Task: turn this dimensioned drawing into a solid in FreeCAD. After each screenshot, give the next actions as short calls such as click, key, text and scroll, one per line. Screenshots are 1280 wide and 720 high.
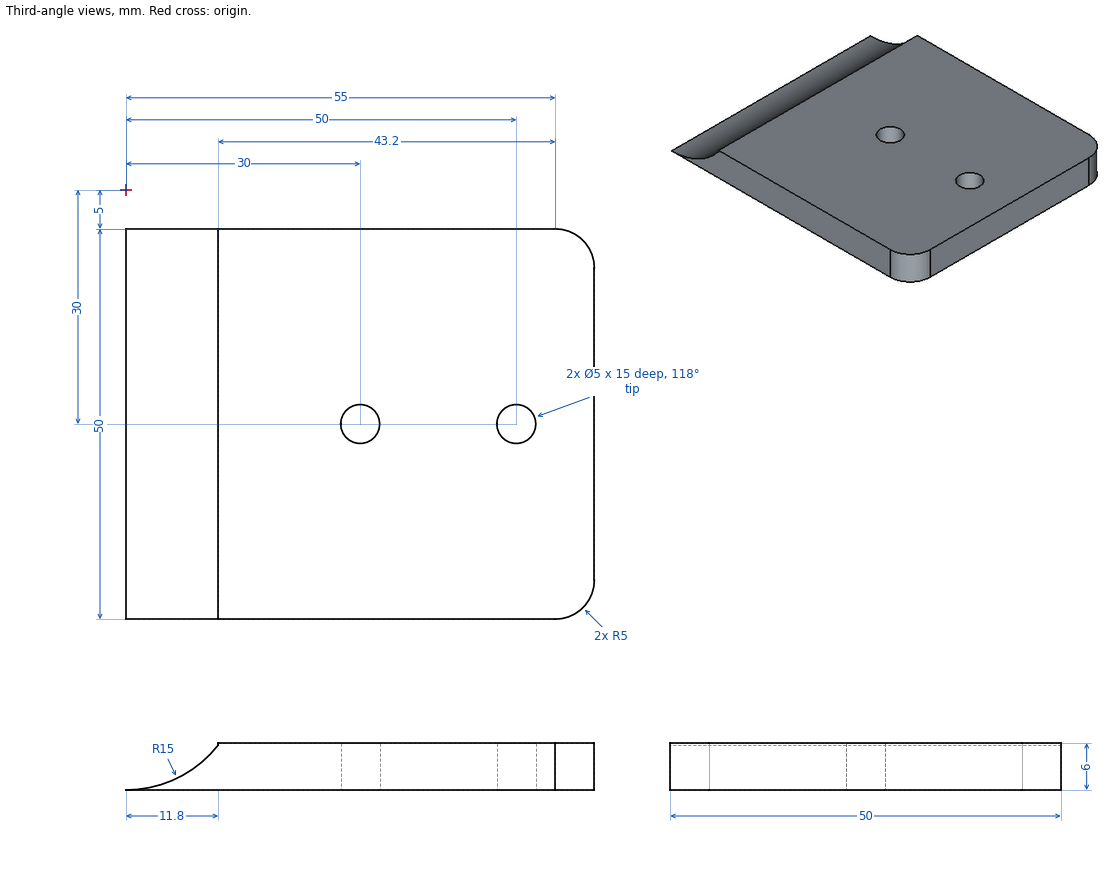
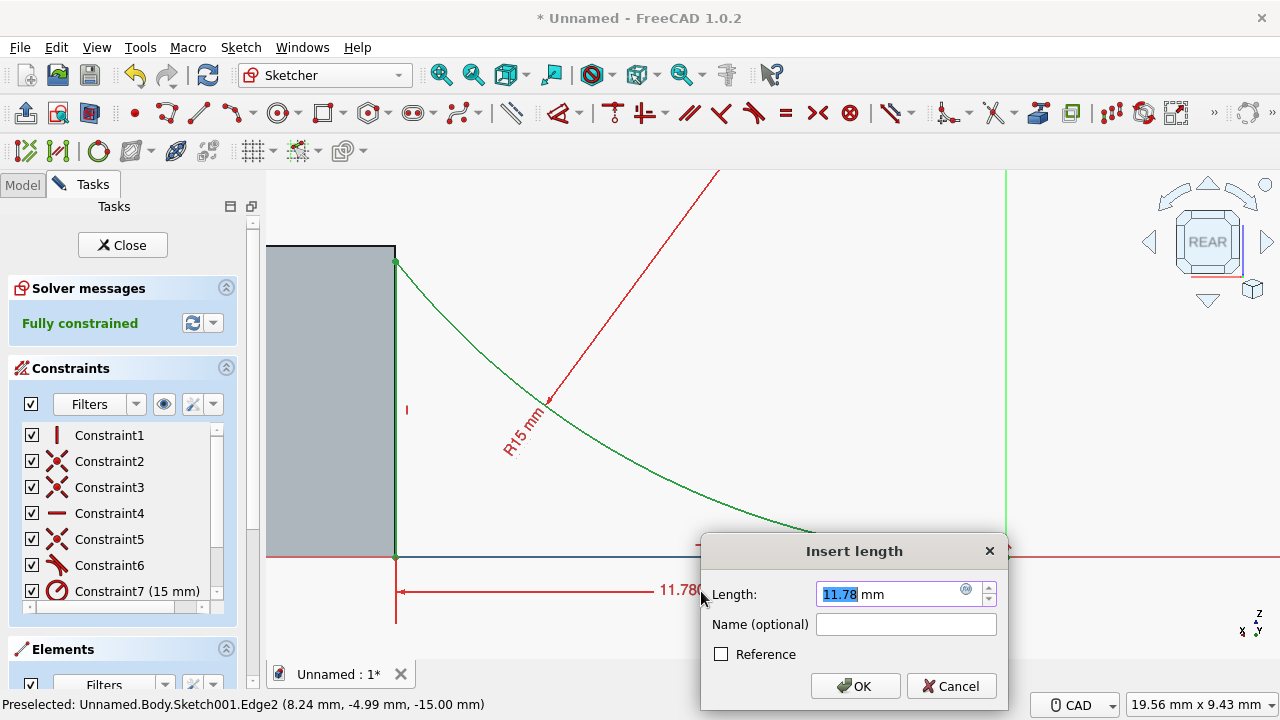
text(11.8)
key(Return)
key(Escape)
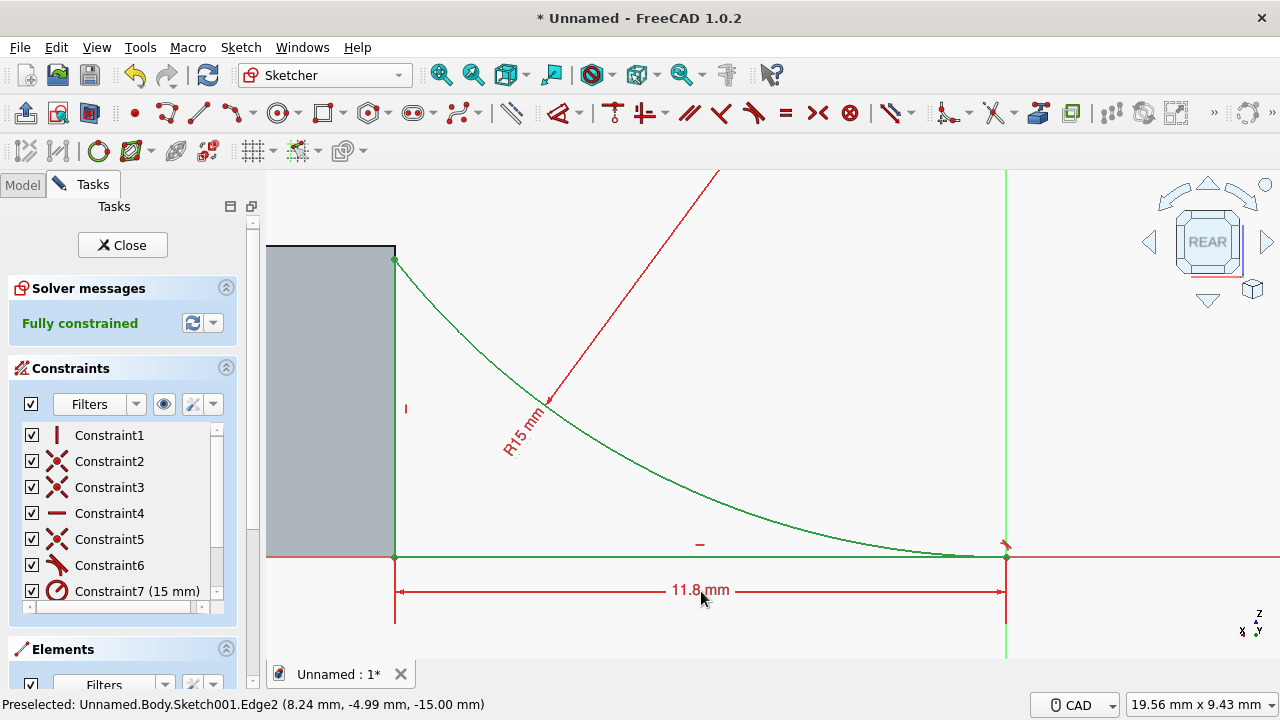
click(123, 245)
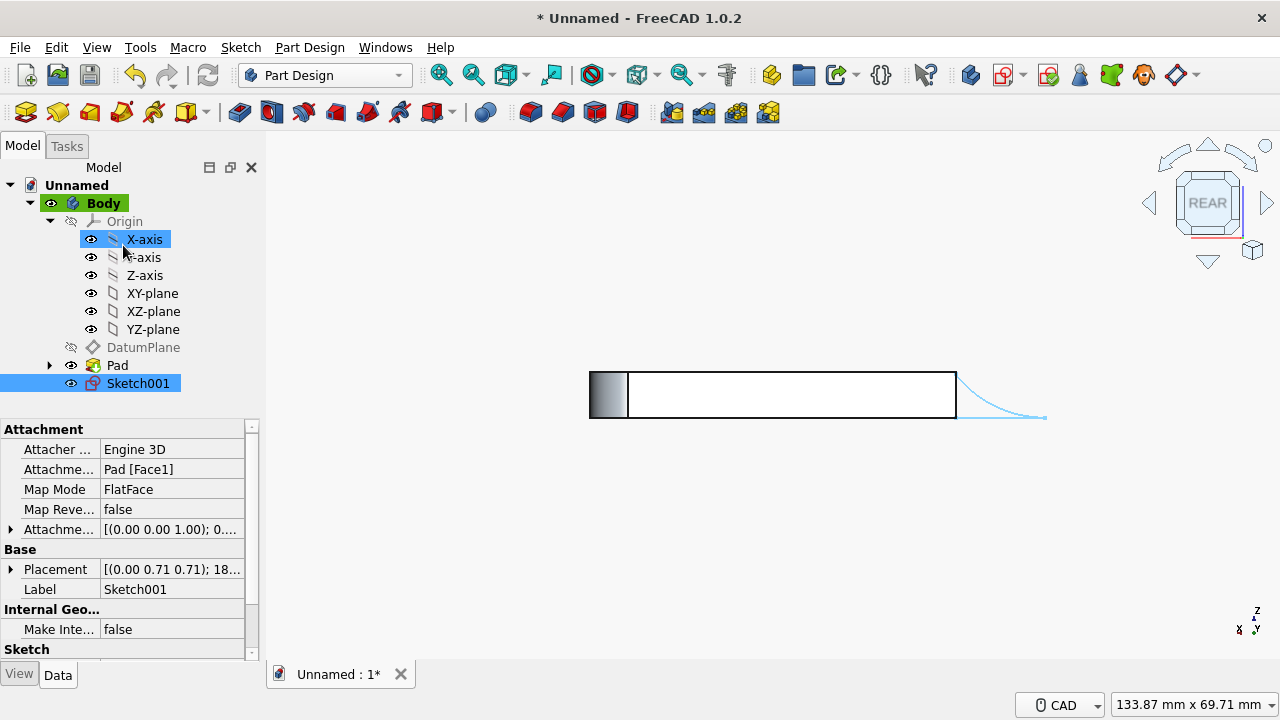
click(26, 112)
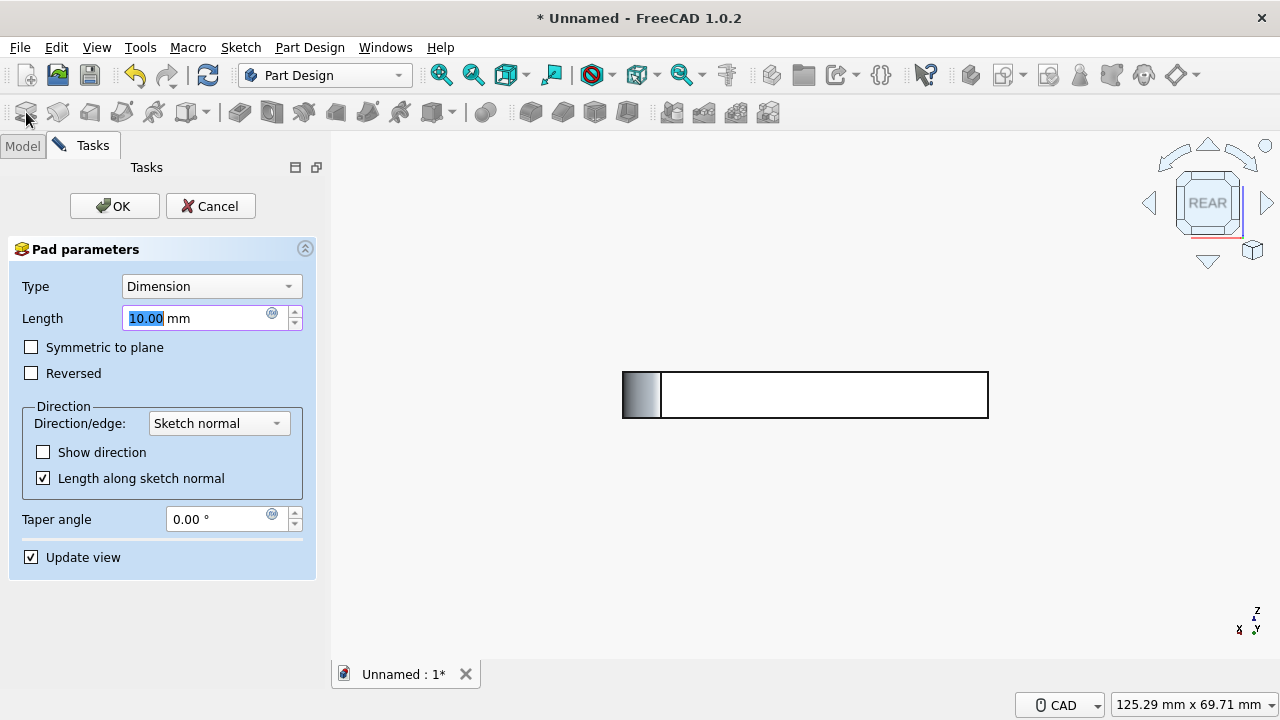
text(50)
key(Tab)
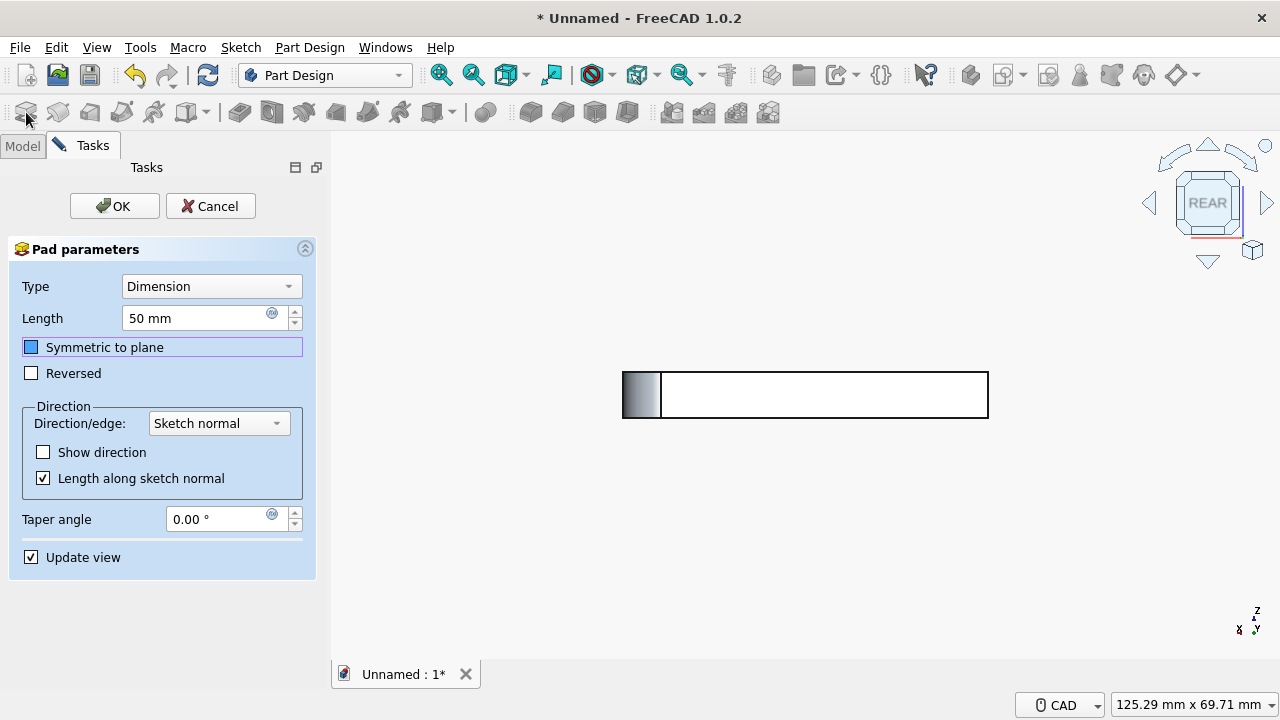
click(30, 373)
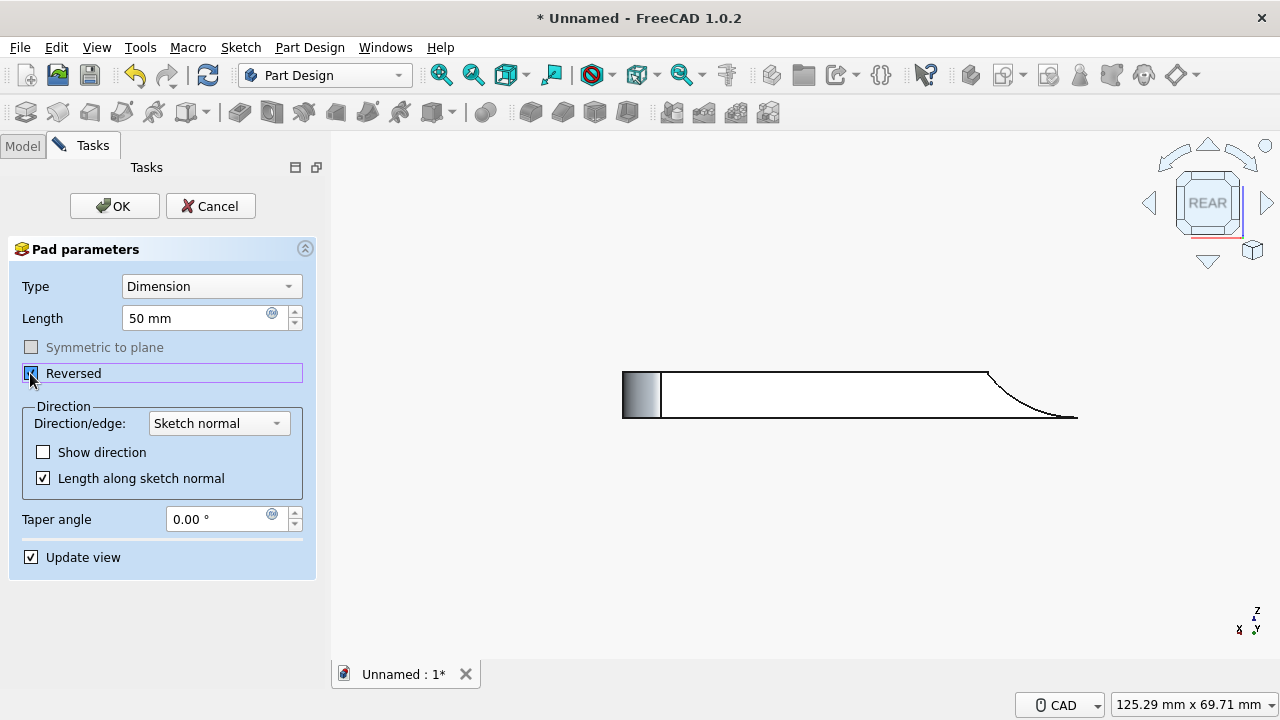
click(115, 206)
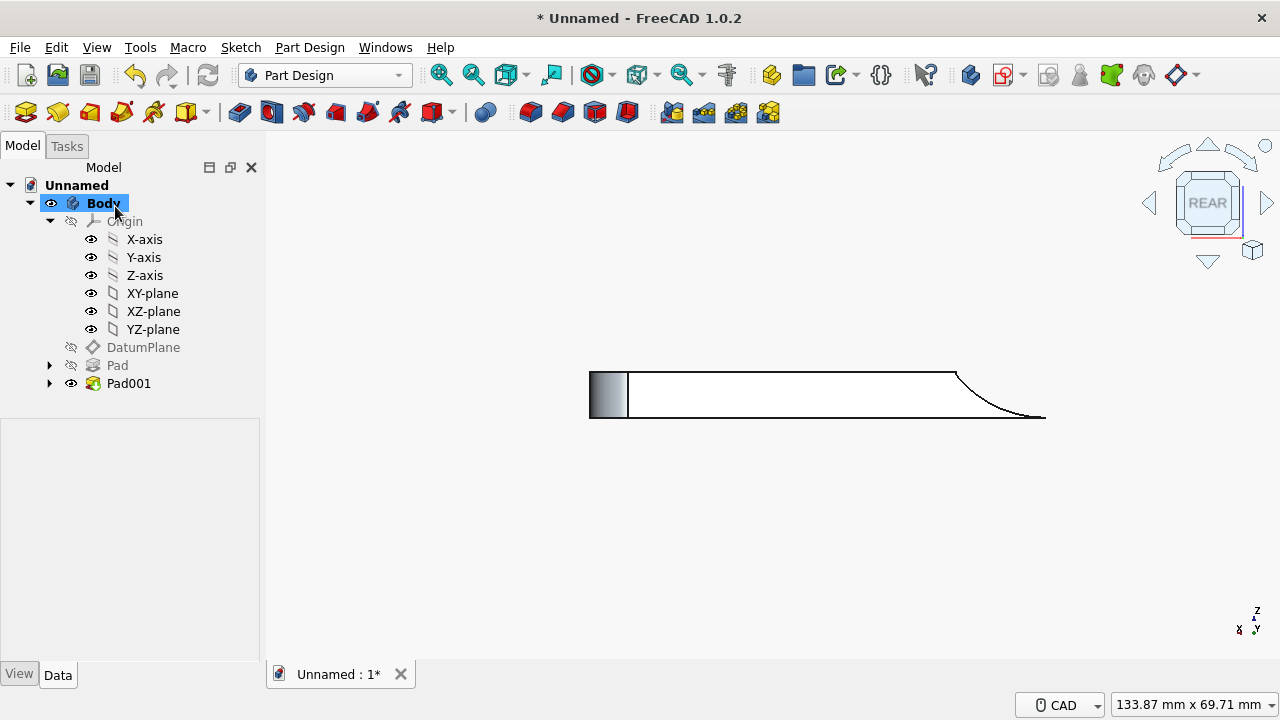
click(442, 76)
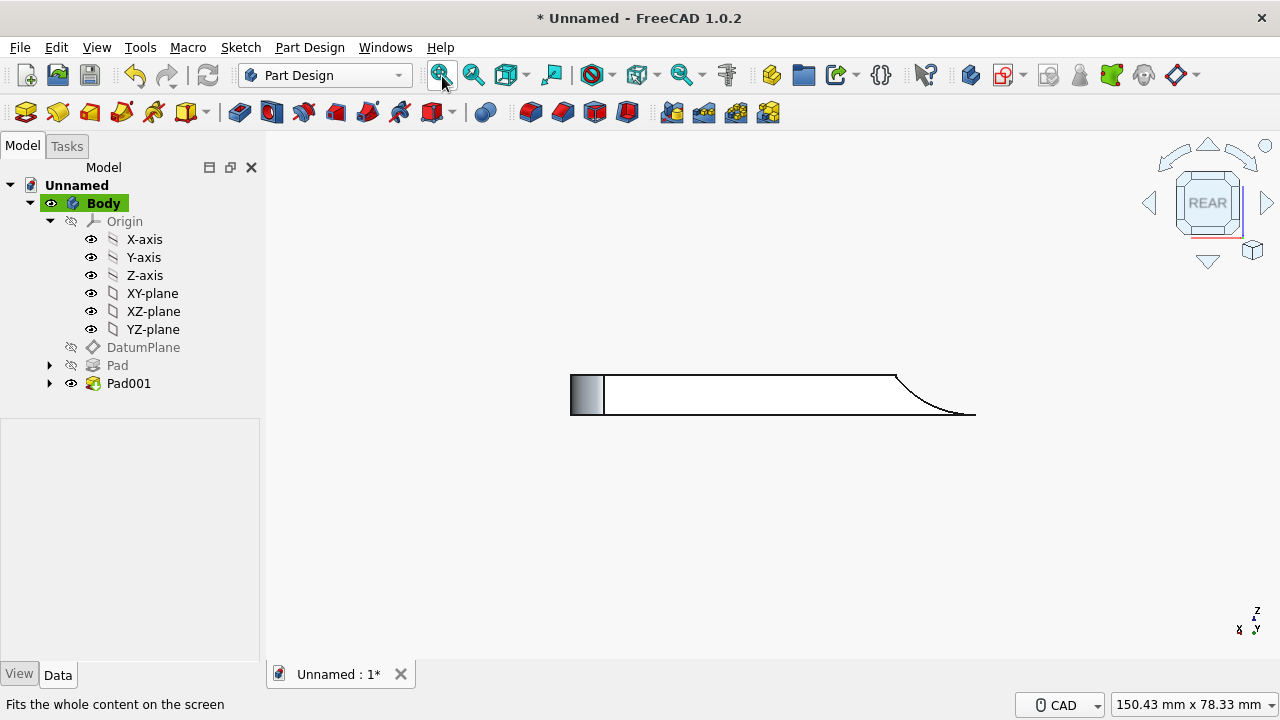
key(0)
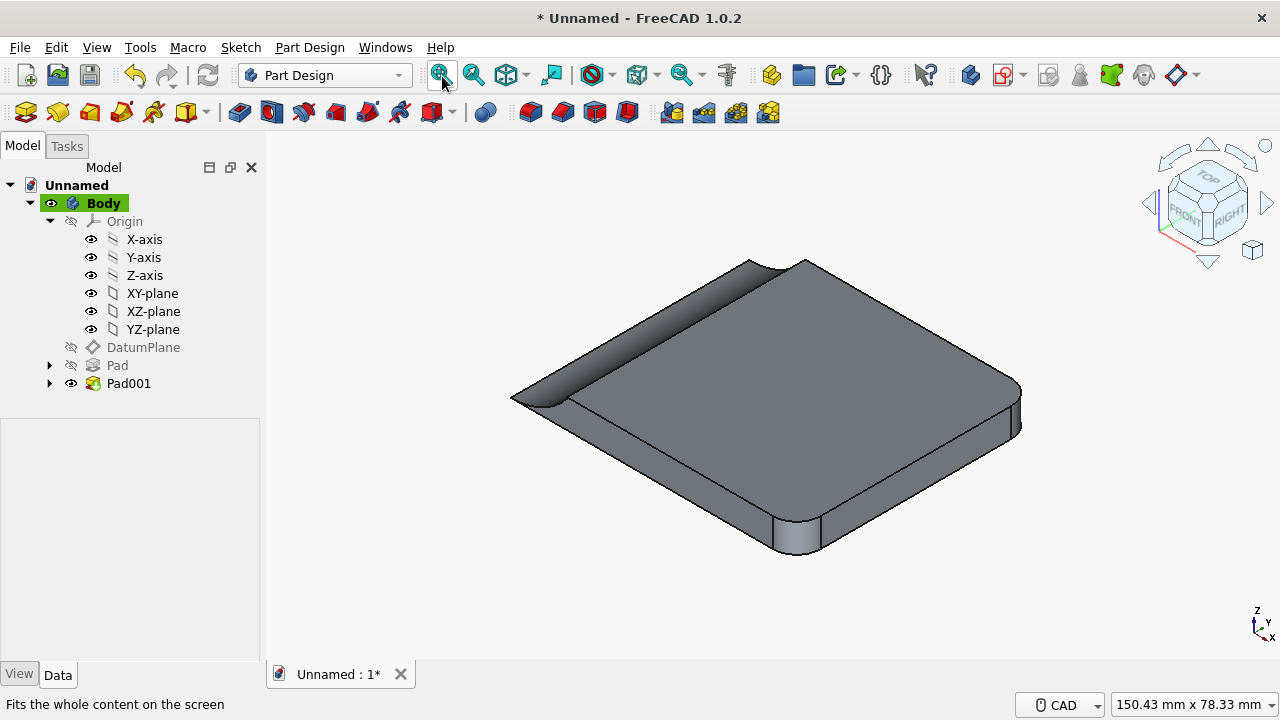
click(801, 394)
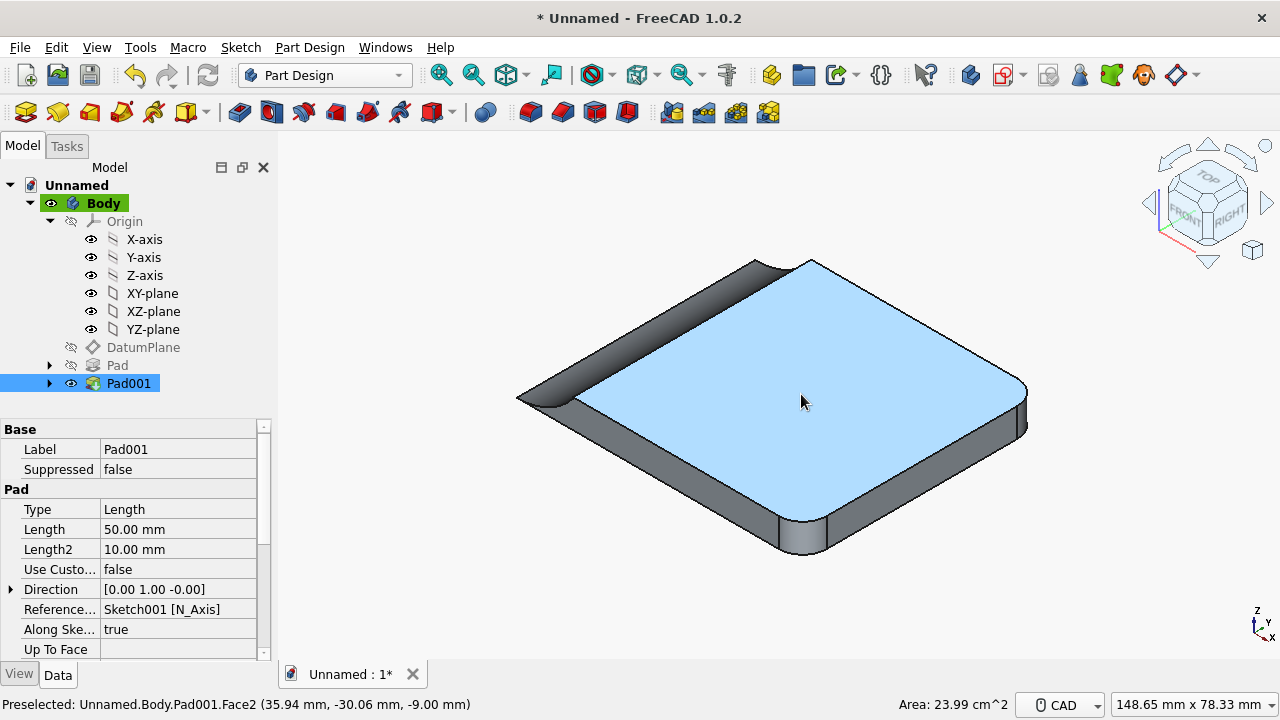
click(1004, 76)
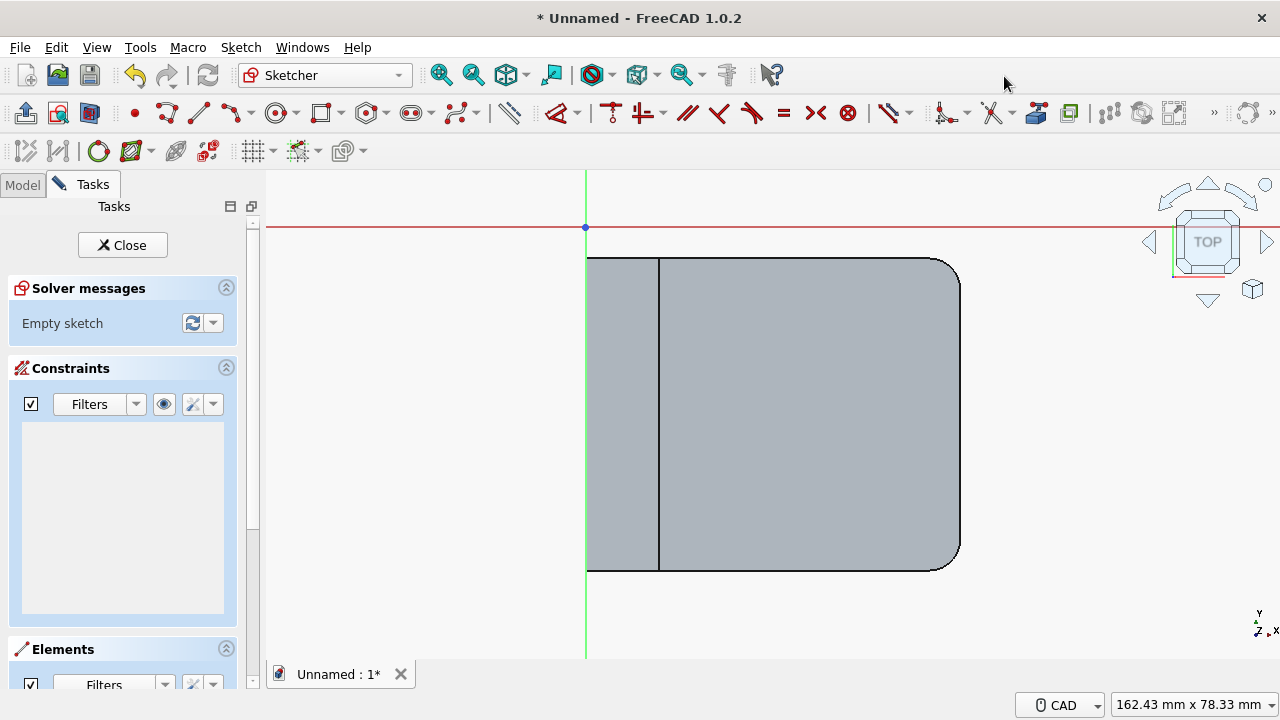
scroll(841, 198, up, 2)